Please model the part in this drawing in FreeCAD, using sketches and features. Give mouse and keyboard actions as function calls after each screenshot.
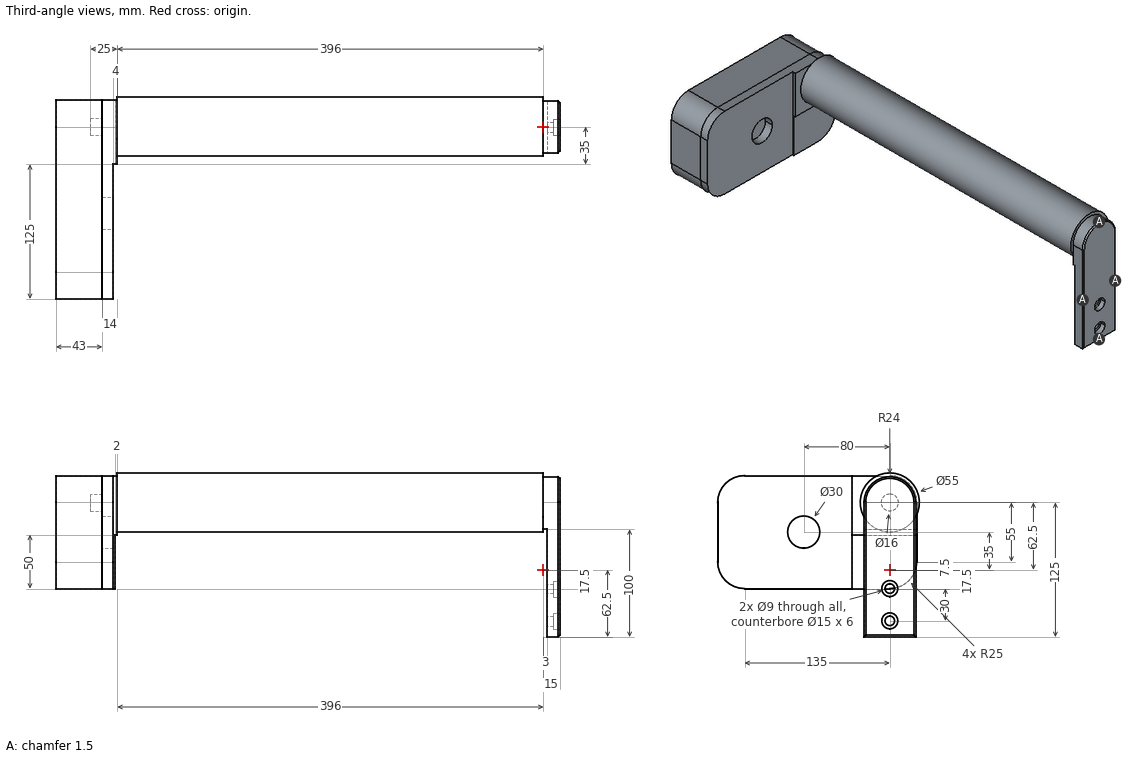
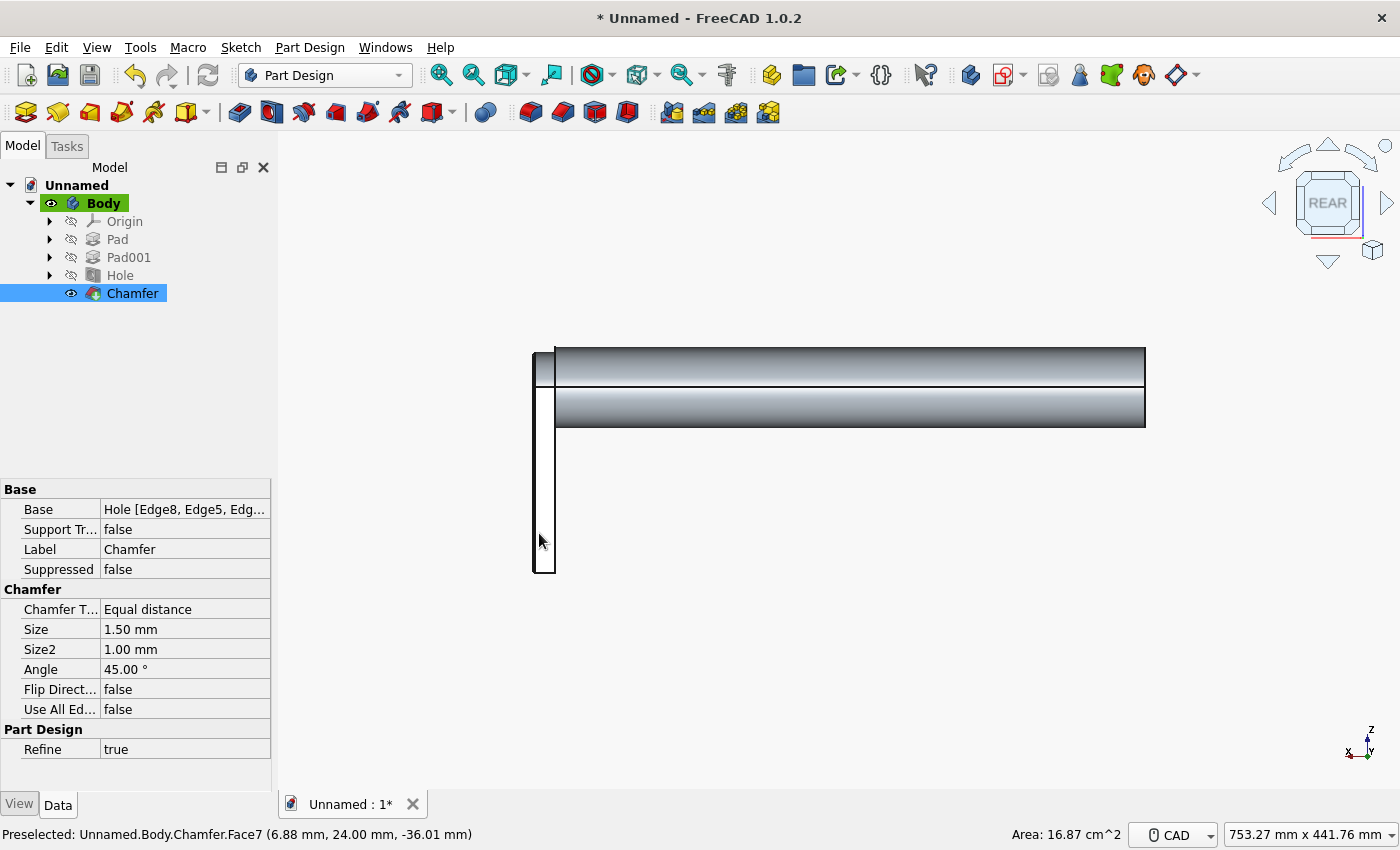
click(1004, 76)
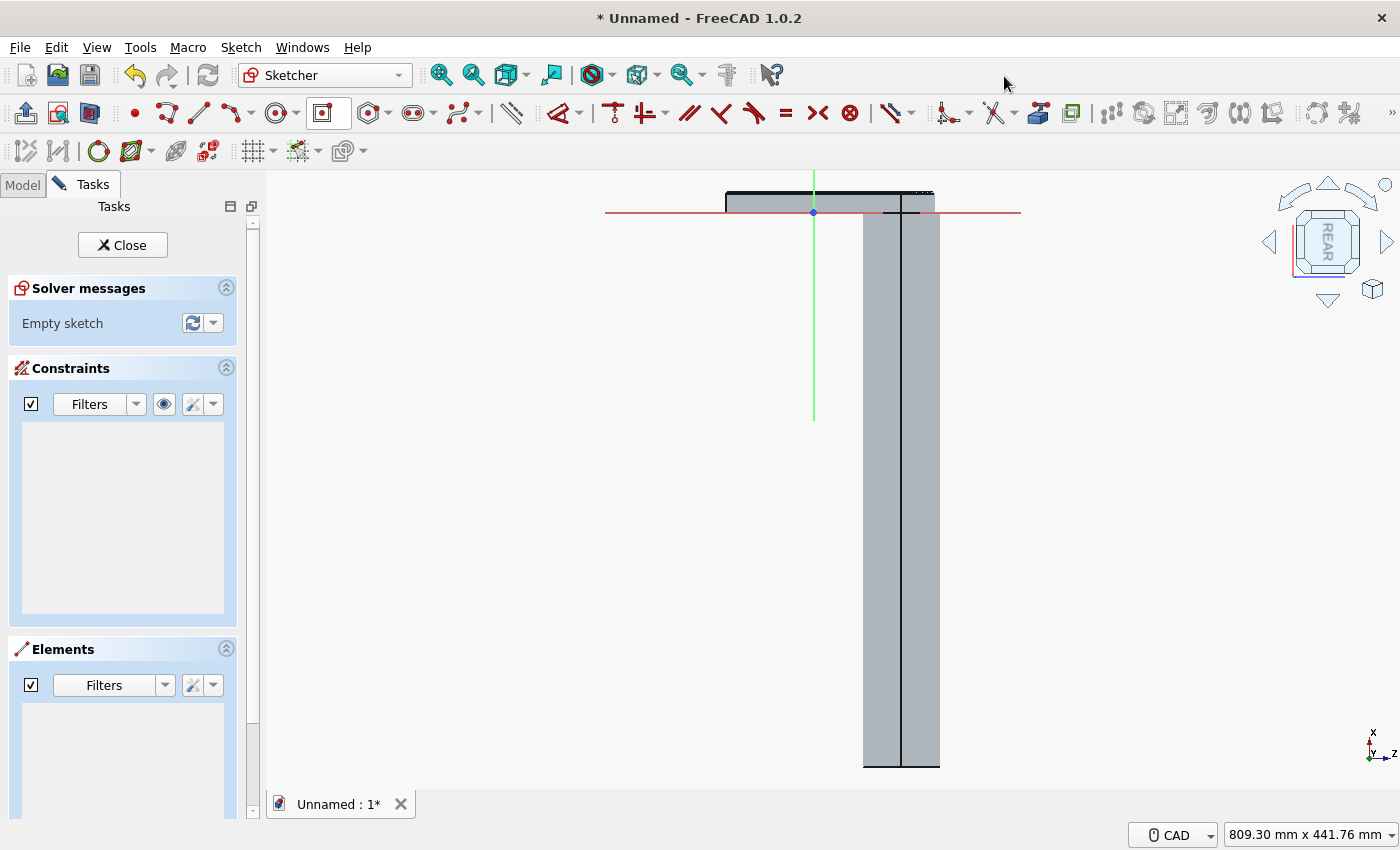
scroll(804, 198, up, 8)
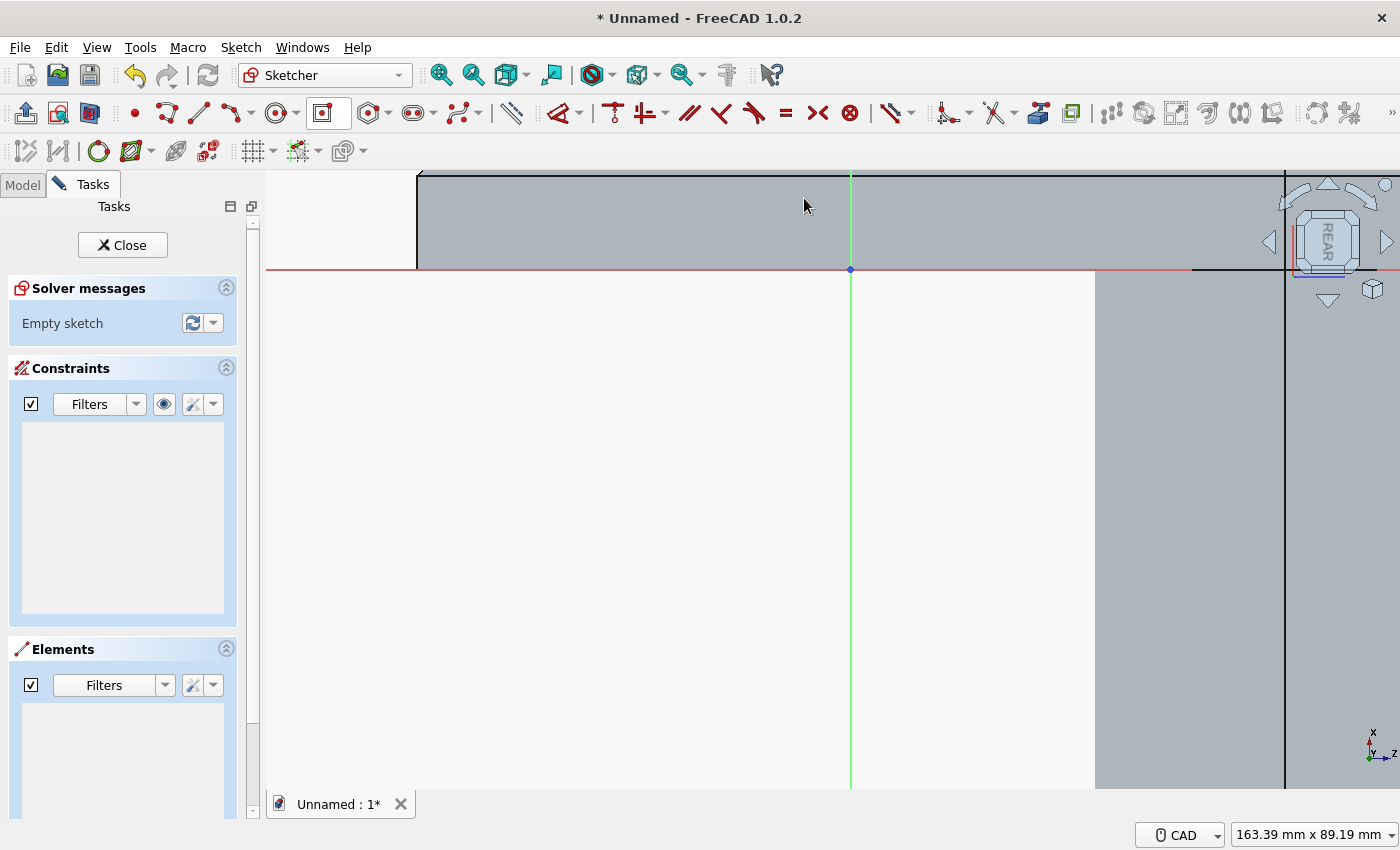
key(g)
key(r)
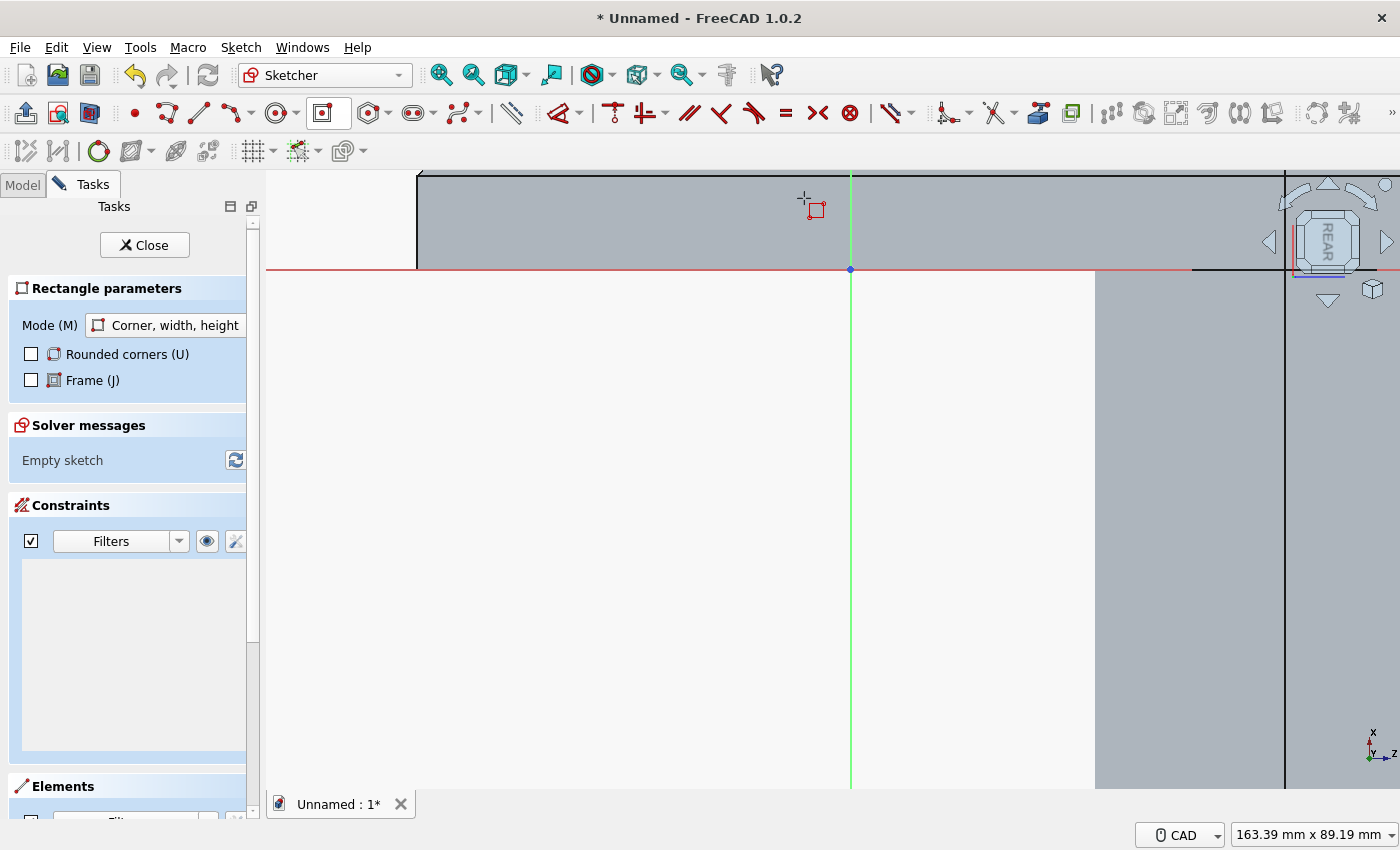
click(417, 249)
click(1111, 270)
key(Escape)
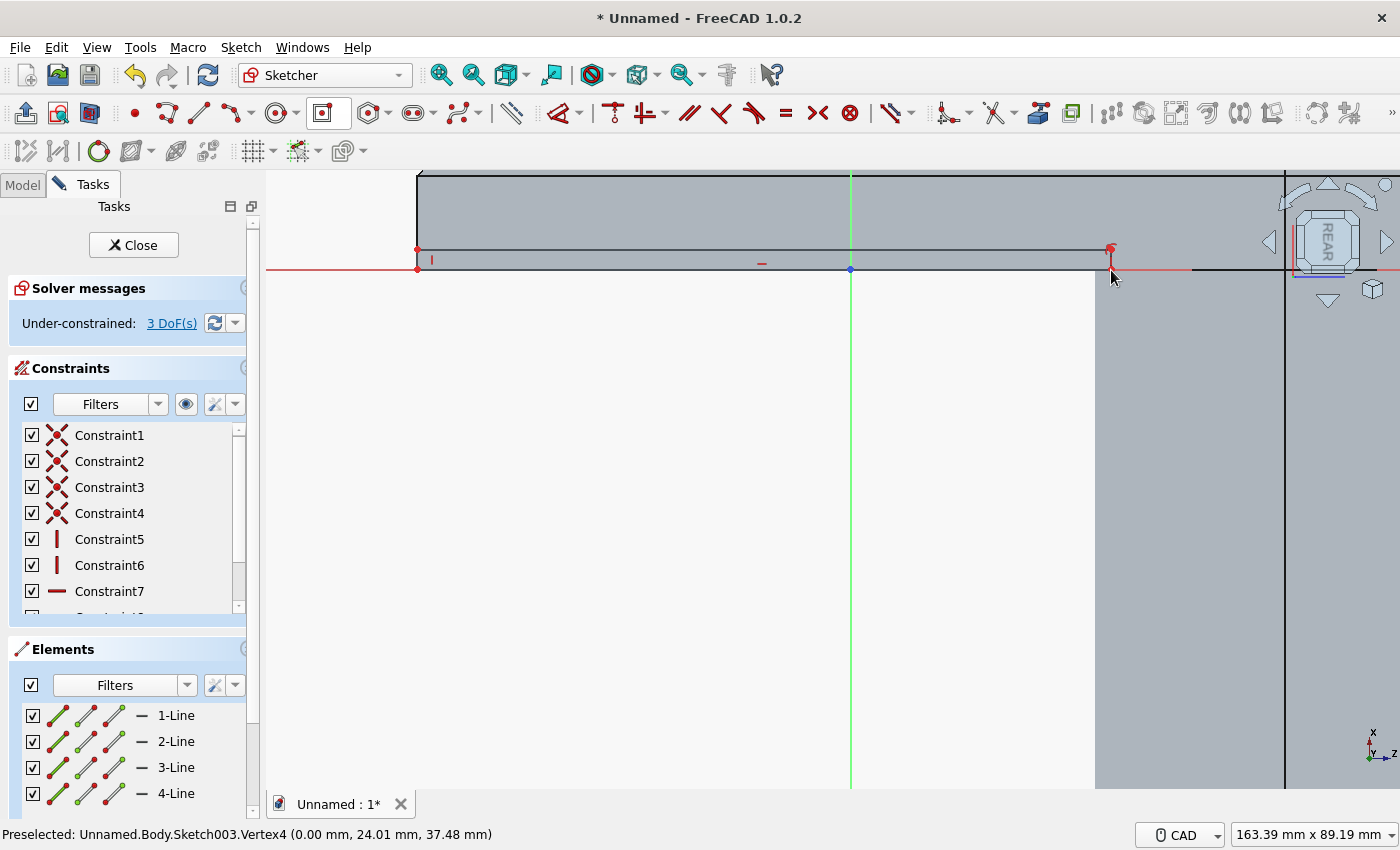
click(558, 114)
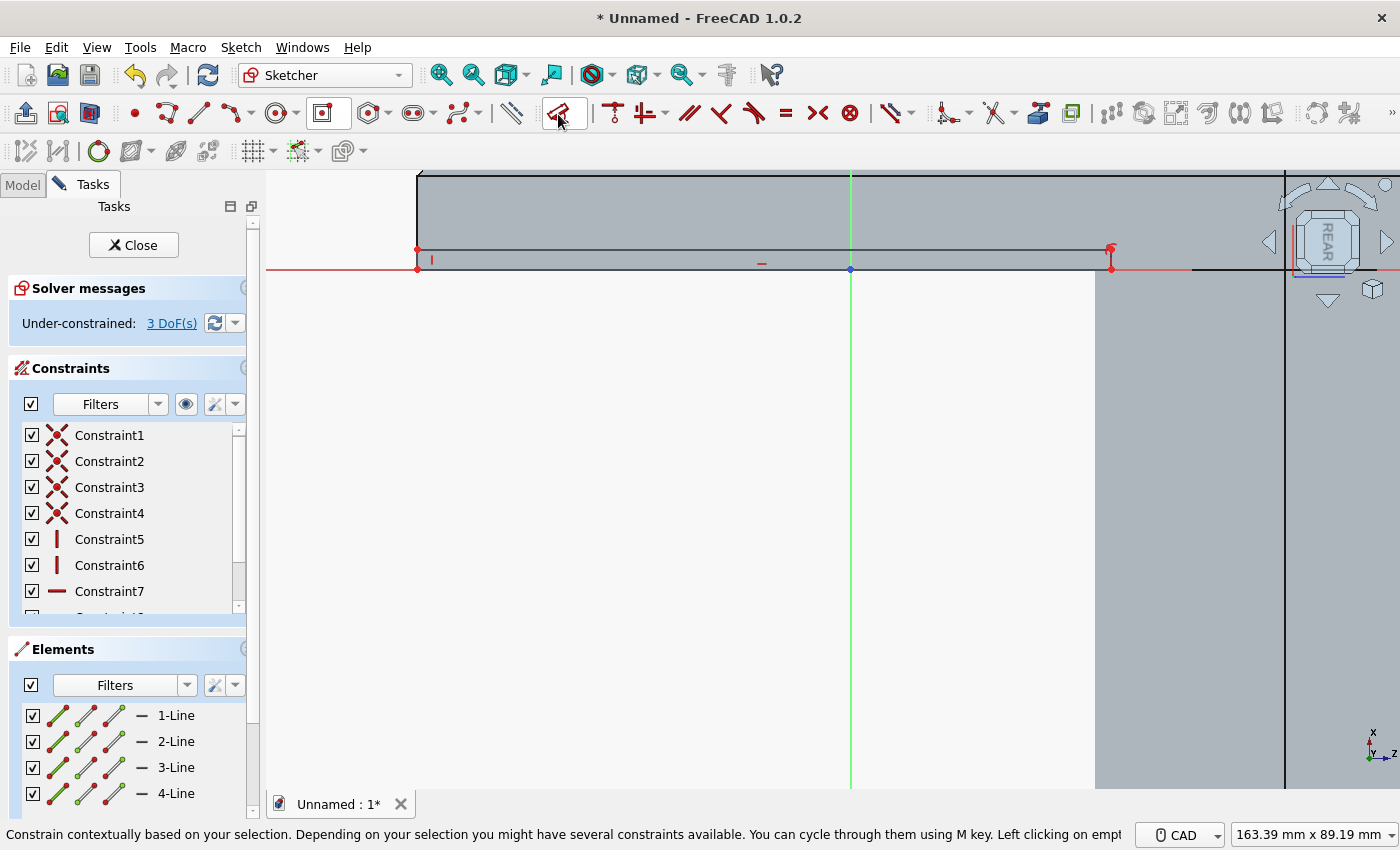
scroll(417, 260, up, 4)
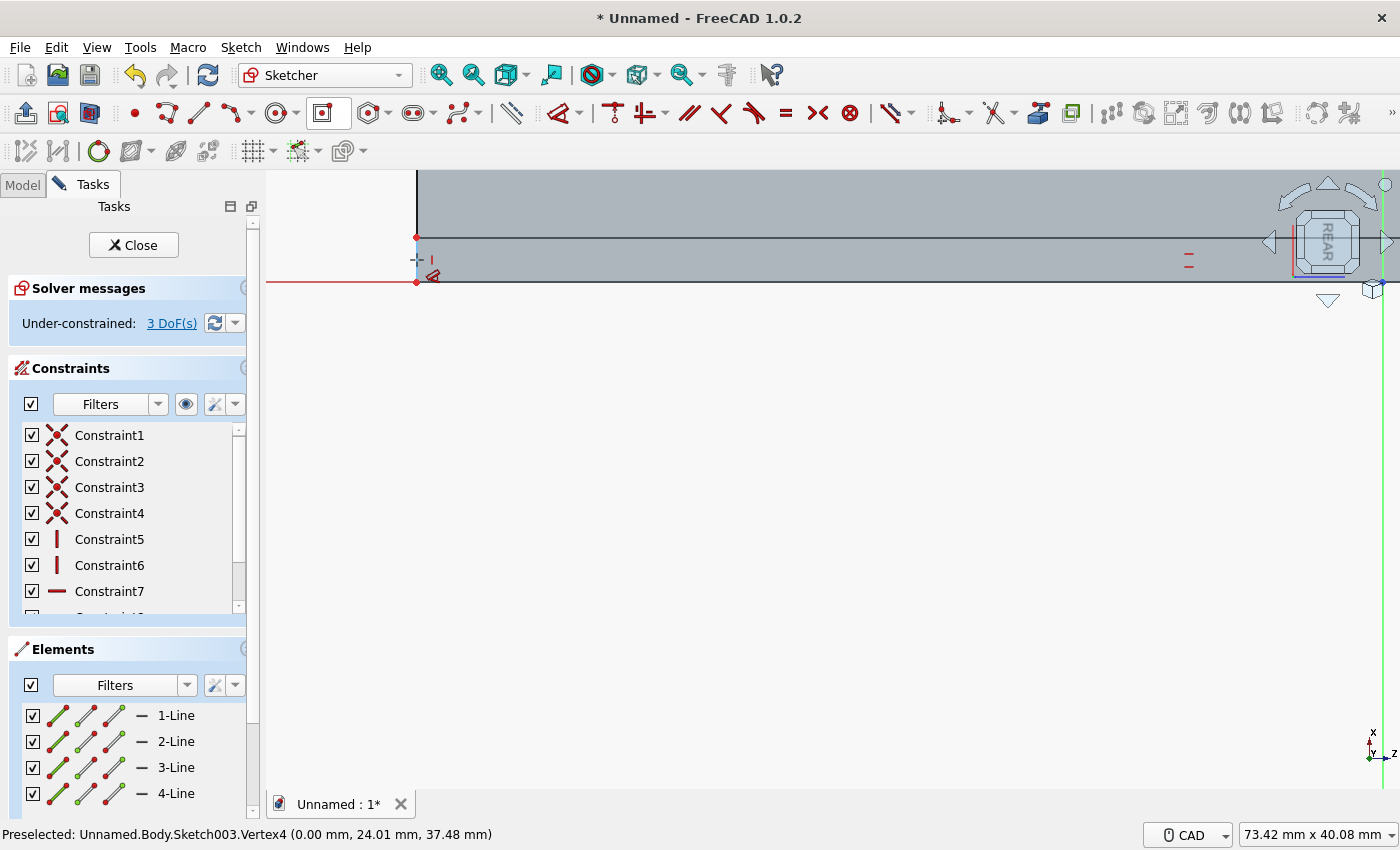
click(417, 260)
click(383, 260)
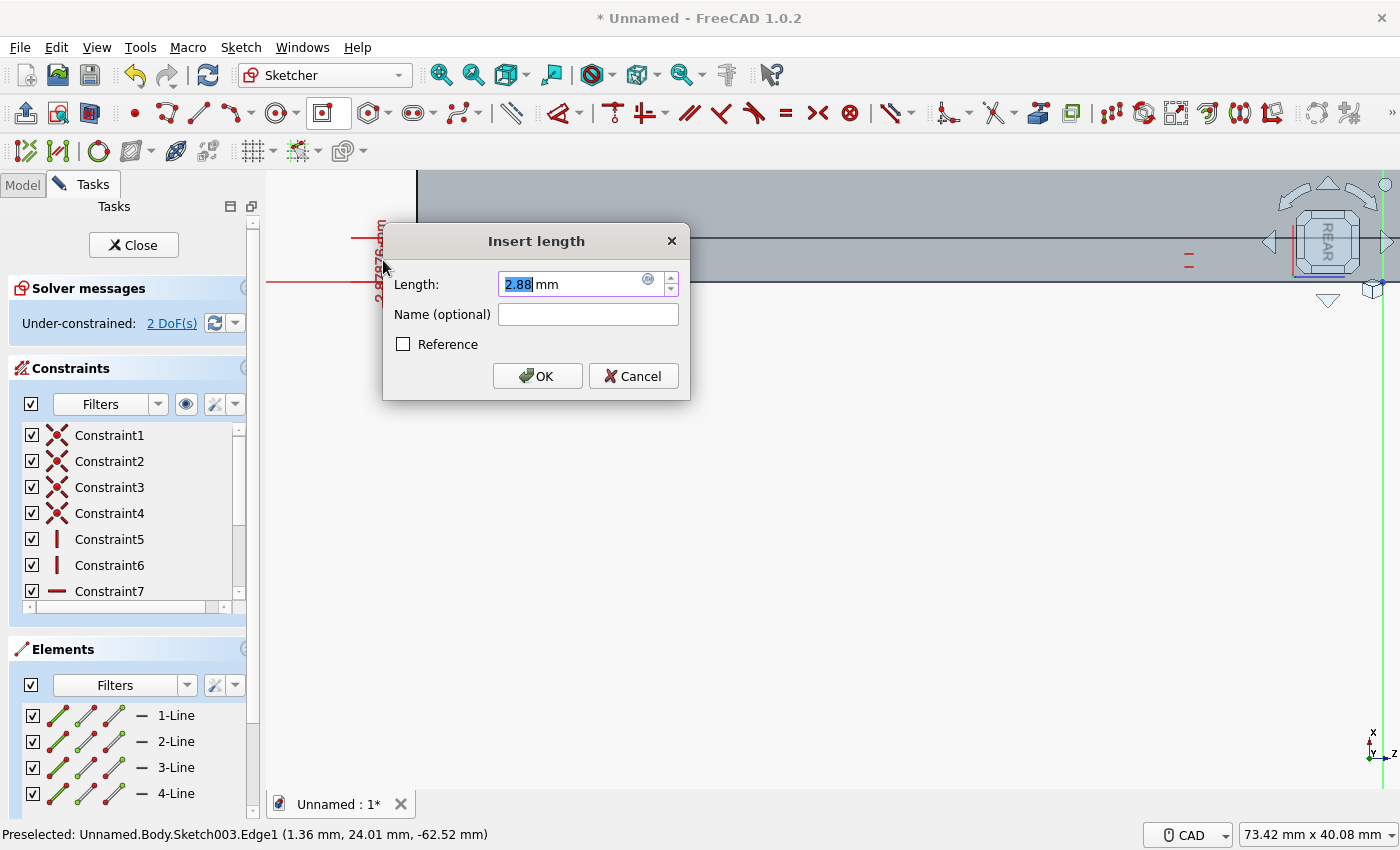
text(3)
key(Return)